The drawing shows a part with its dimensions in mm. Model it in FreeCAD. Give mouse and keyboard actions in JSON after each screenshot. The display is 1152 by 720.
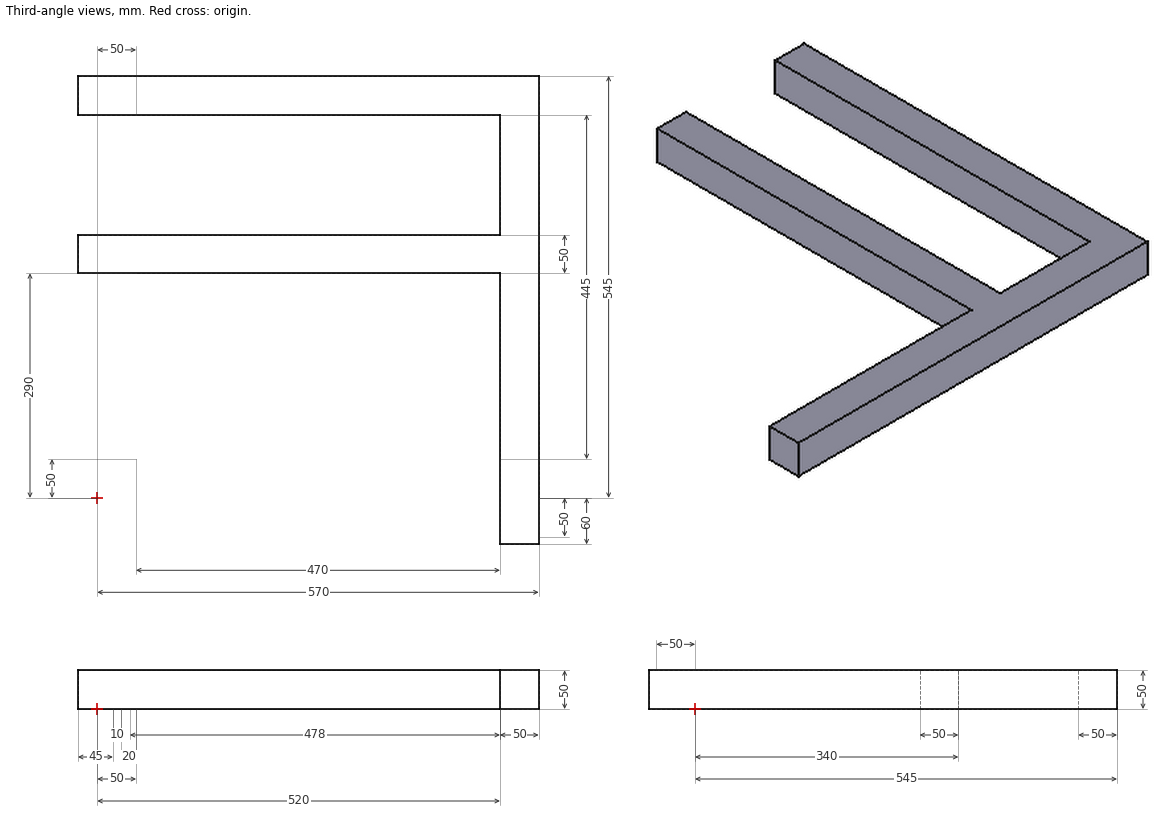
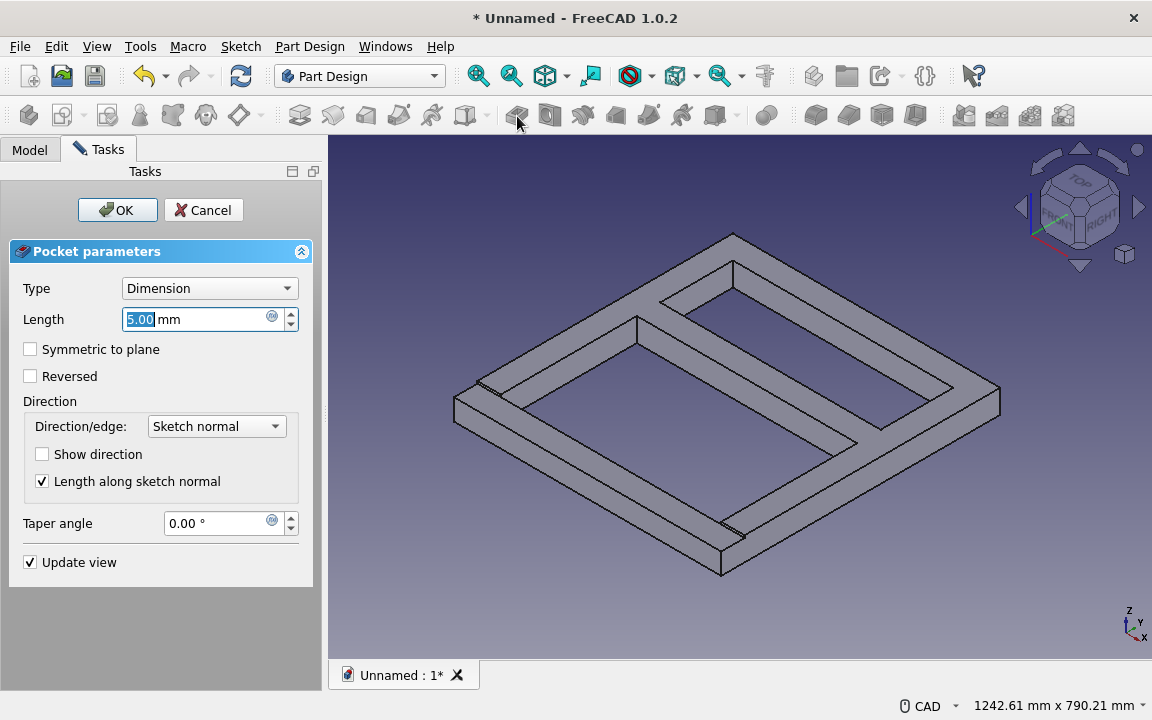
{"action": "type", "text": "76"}
{"action": "key", "text": "Tab"}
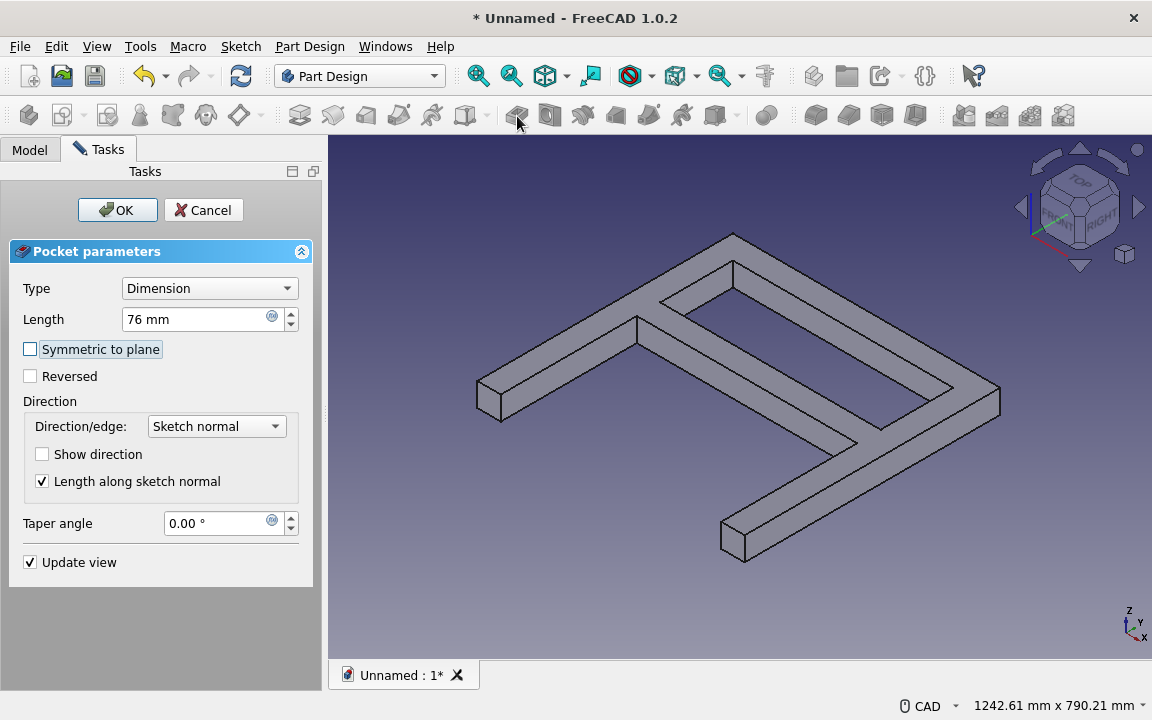
{"action": "left_click", "coordinate": [118, 210]}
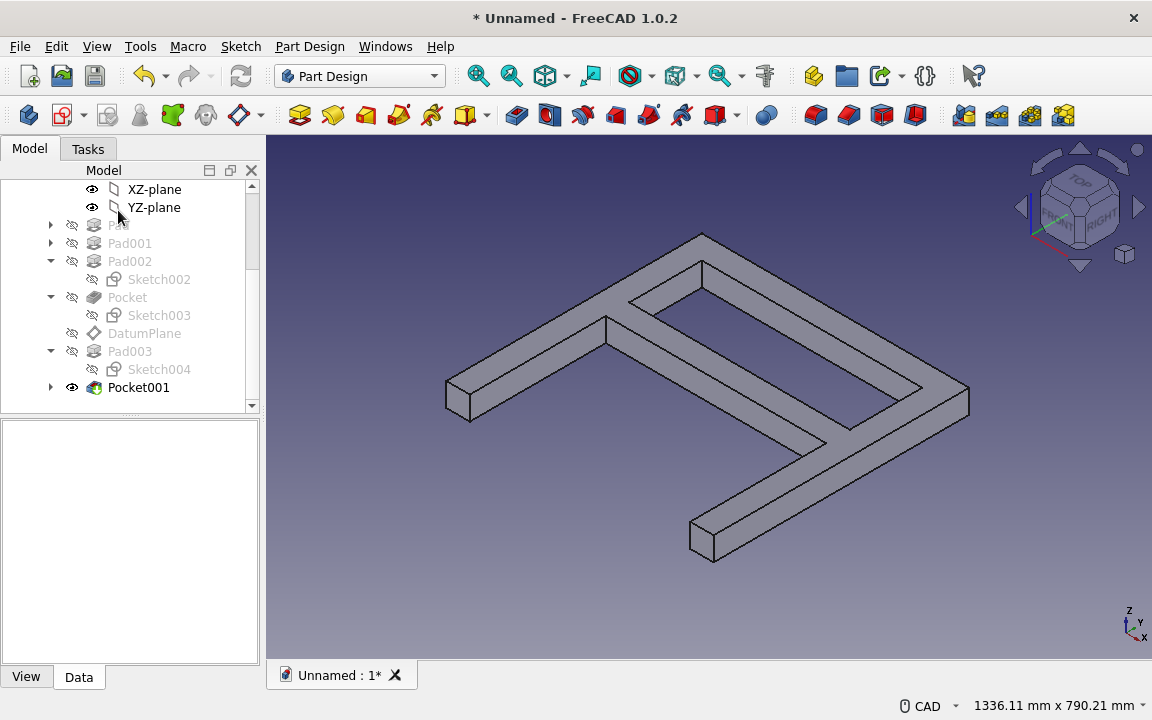
{"action": "left_click", "coordinate": [62, 116]}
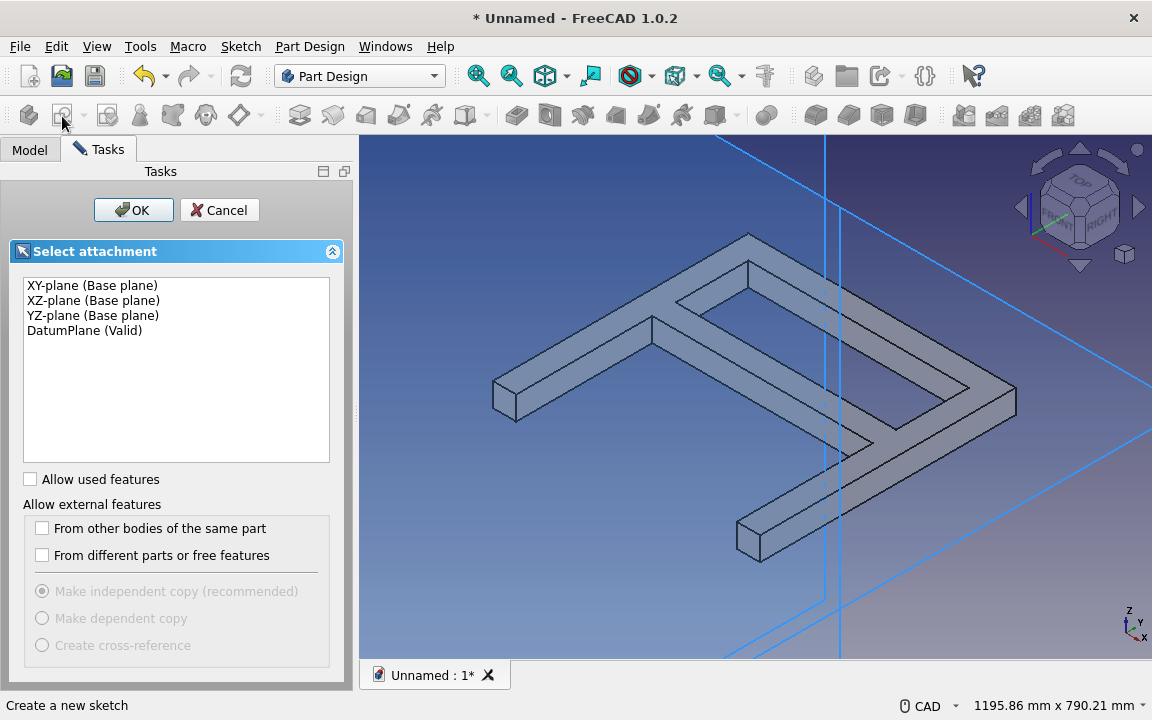
{"action": "left_click", "coordinate": [84, 316]}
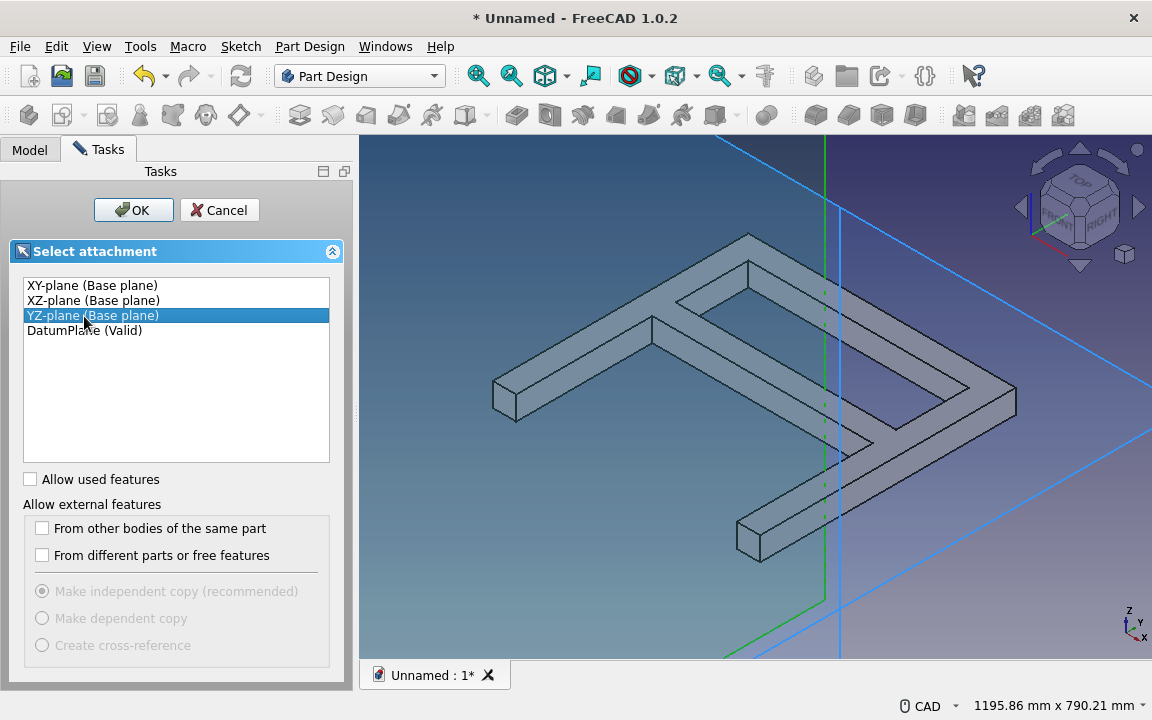
{"action": "left_click", "coordinate": [134, 210]}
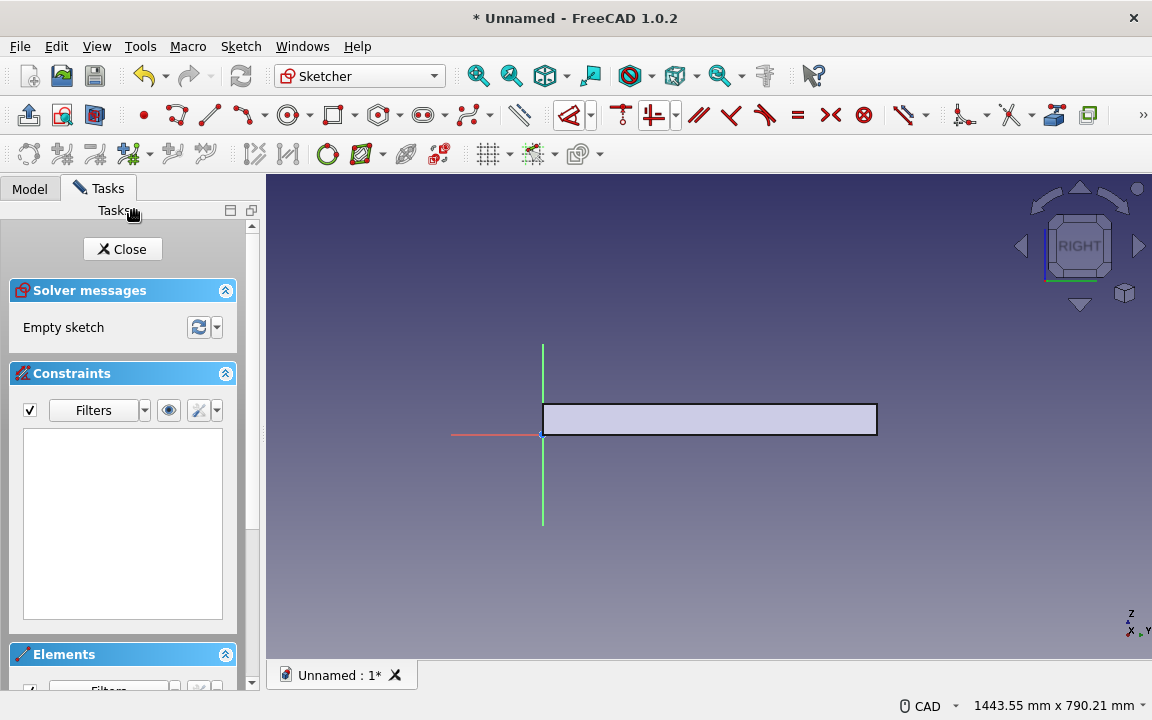
{"action": "key", "text": "q s"}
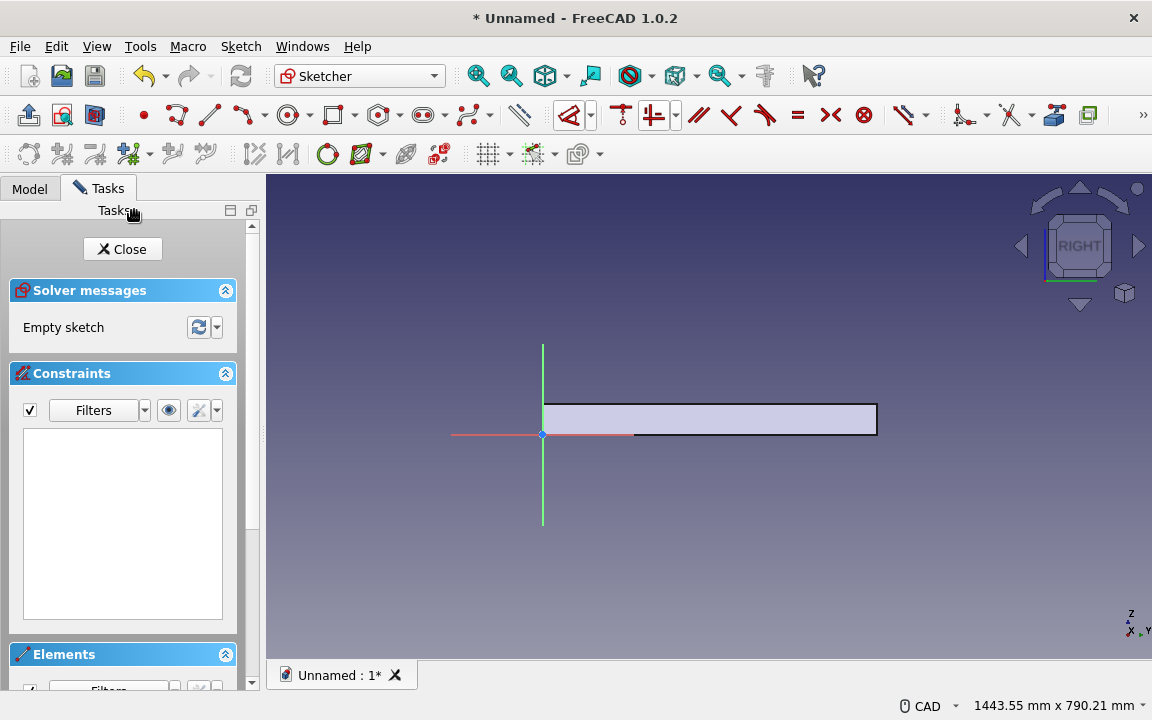
{"action": "scroll", "coordinate": [852, 425], "scroll_direction": "up", "scroll_amount": 2}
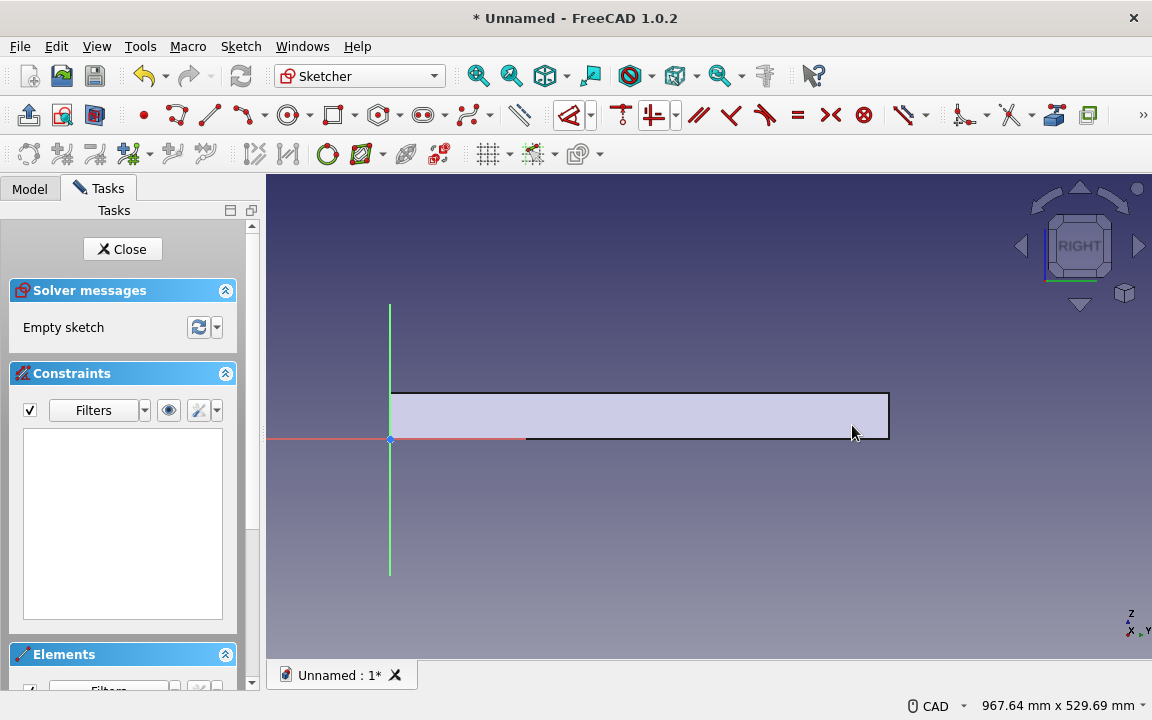
{"action": "key", "text": "g r"}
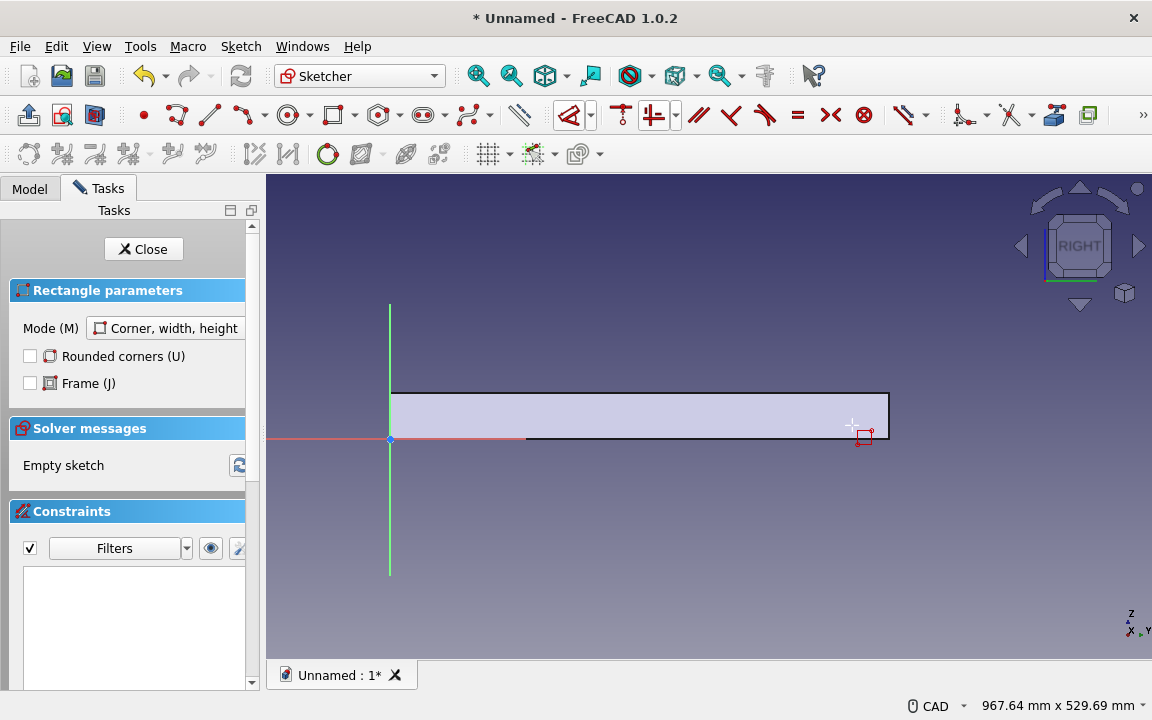
{"action": "left_click", "coordinate": [390, 439]}
{"action": "mouse_move", "coordinate": [889, 393]}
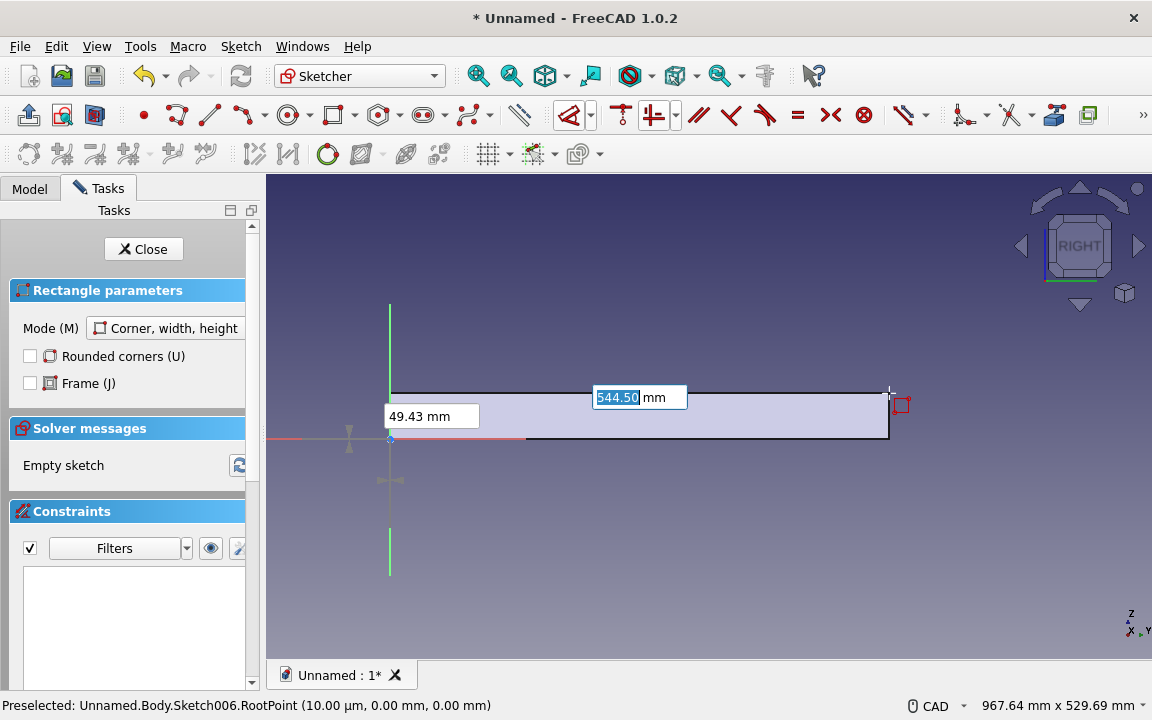
{"action": "type", "text": "545"}
{"action": "key", "text": "Tab"}
{"action": "type", "text": "50"}
{"action": "key", "text": "Return"}
{"action": "key", "text": "Escape"}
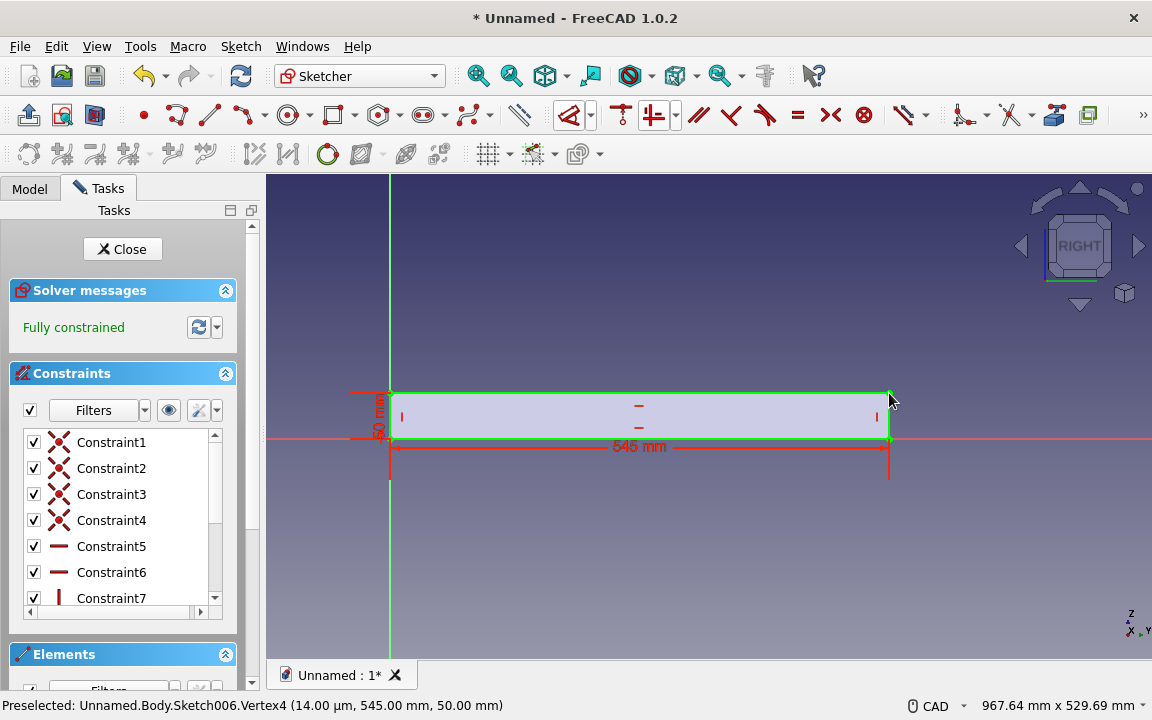
{"action": "left_click", "coordinate": [123, 249]}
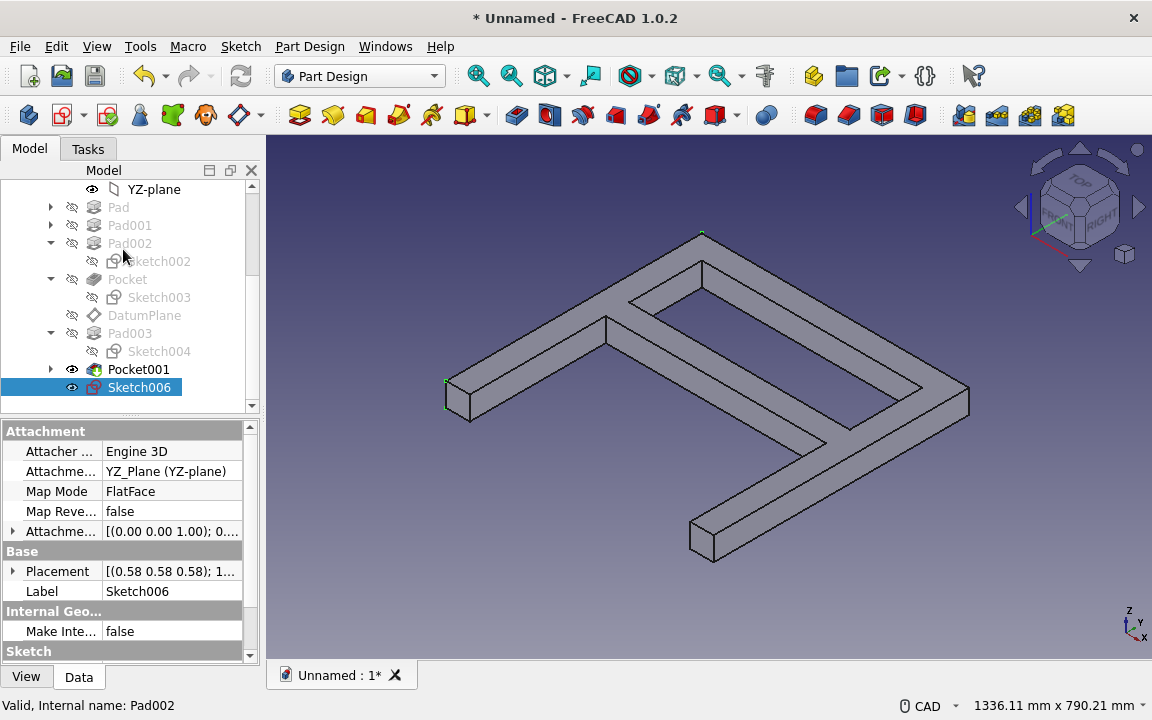
{"action": "left_click", "coordinate": [517, 116]}